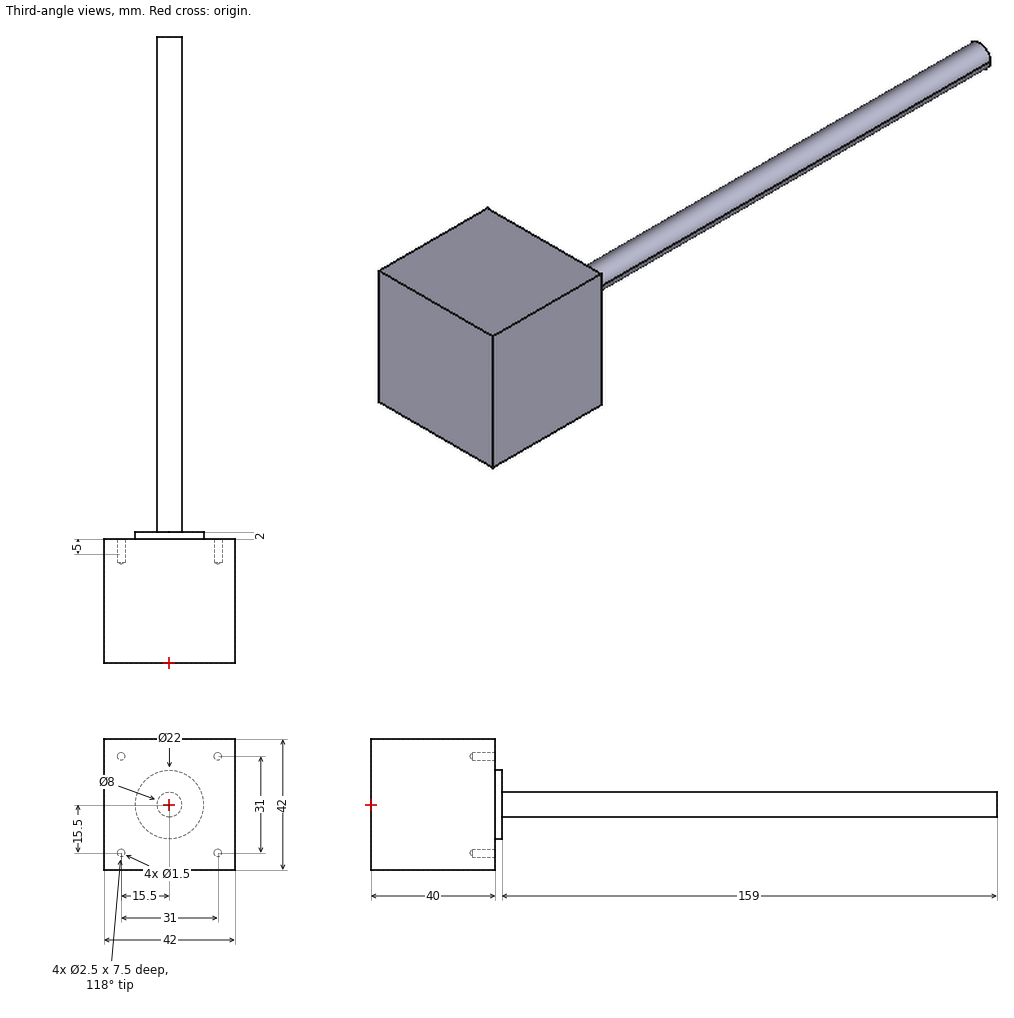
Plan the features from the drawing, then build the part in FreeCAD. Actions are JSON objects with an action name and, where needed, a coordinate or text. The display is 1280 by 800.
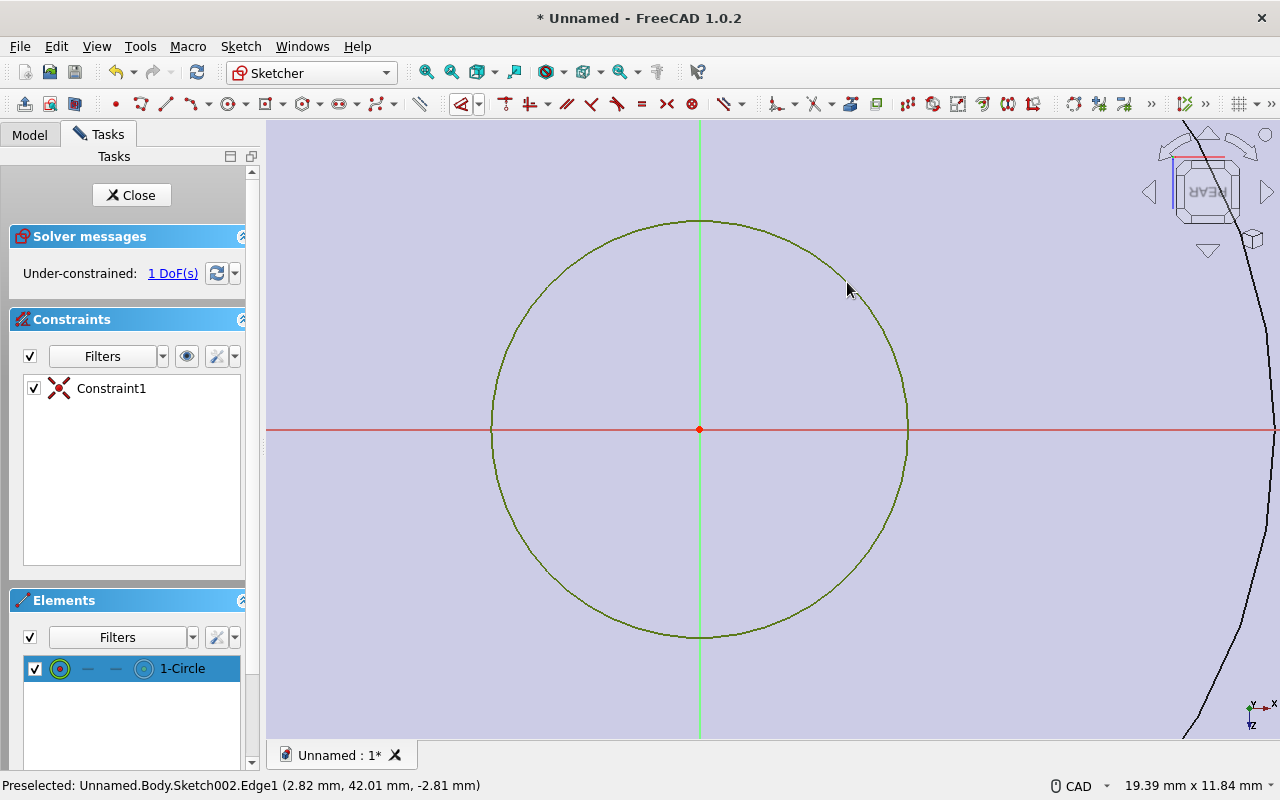
{"action": "key", "text": "k o"}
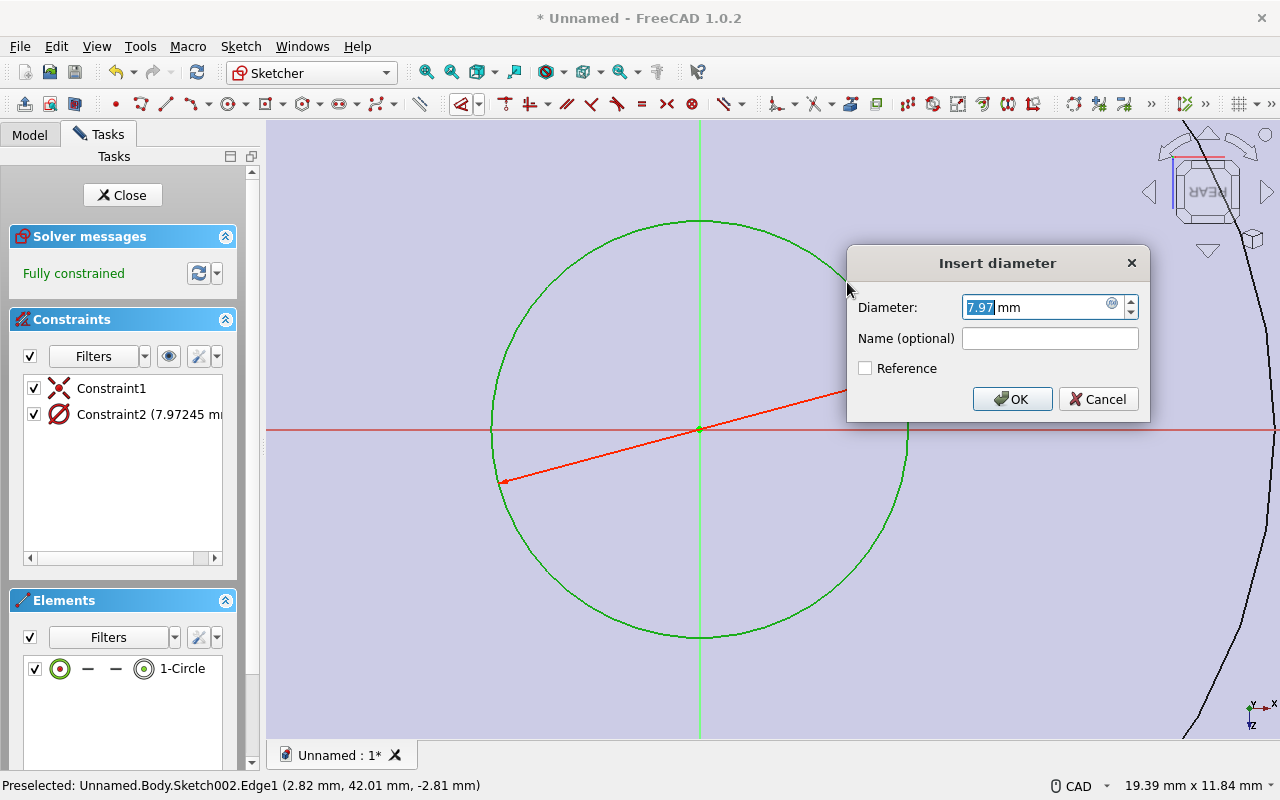
{"action": "type", "text": "8"}
{"action": "key", "text": "Return"}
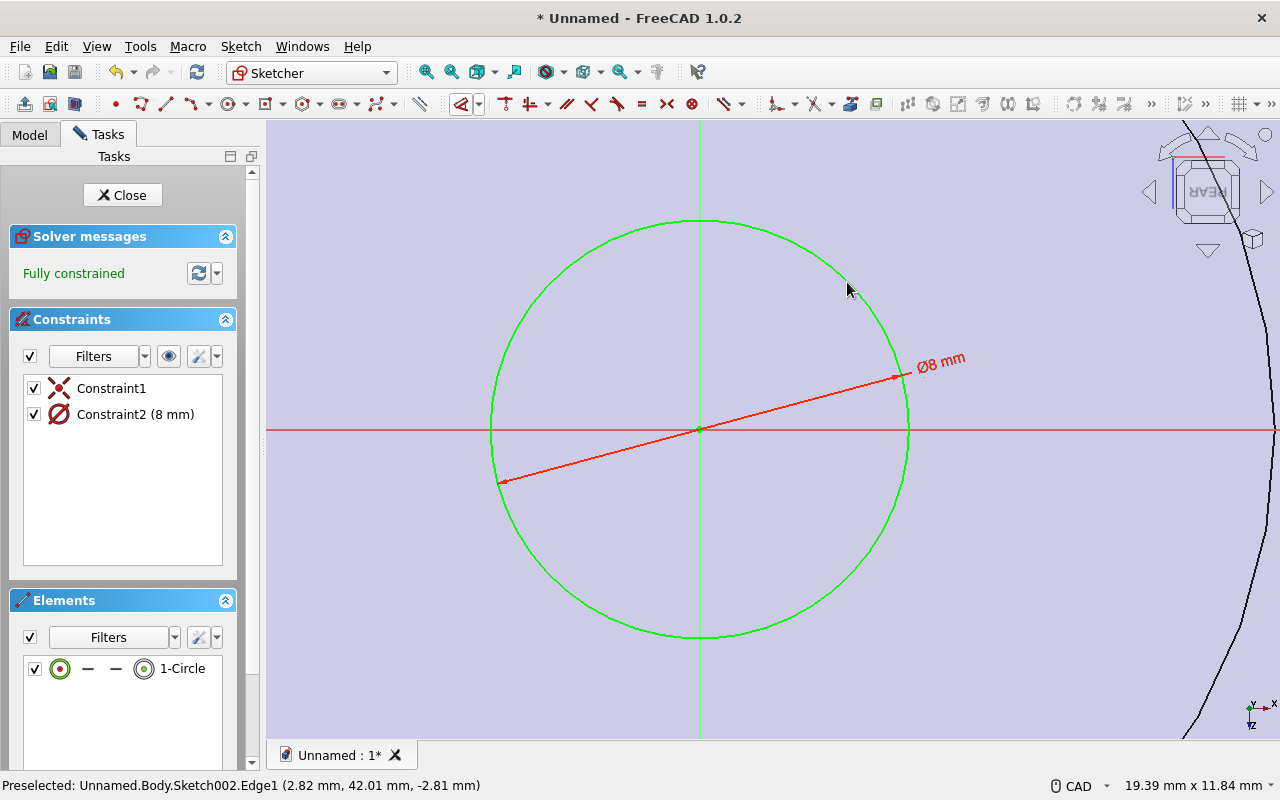
{"action": "left_click", "coordinate": [123, 195]}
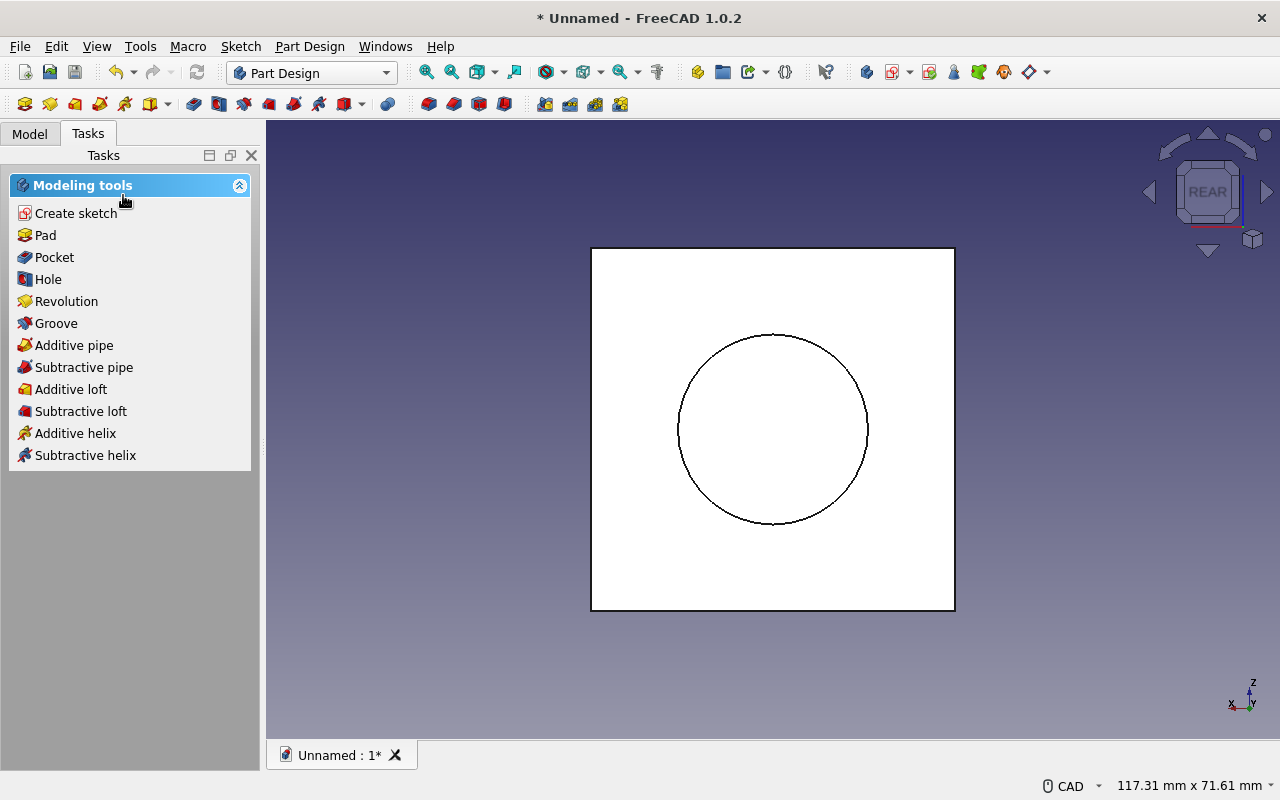
{"action": "left_click", "coordinate": [25, 104]}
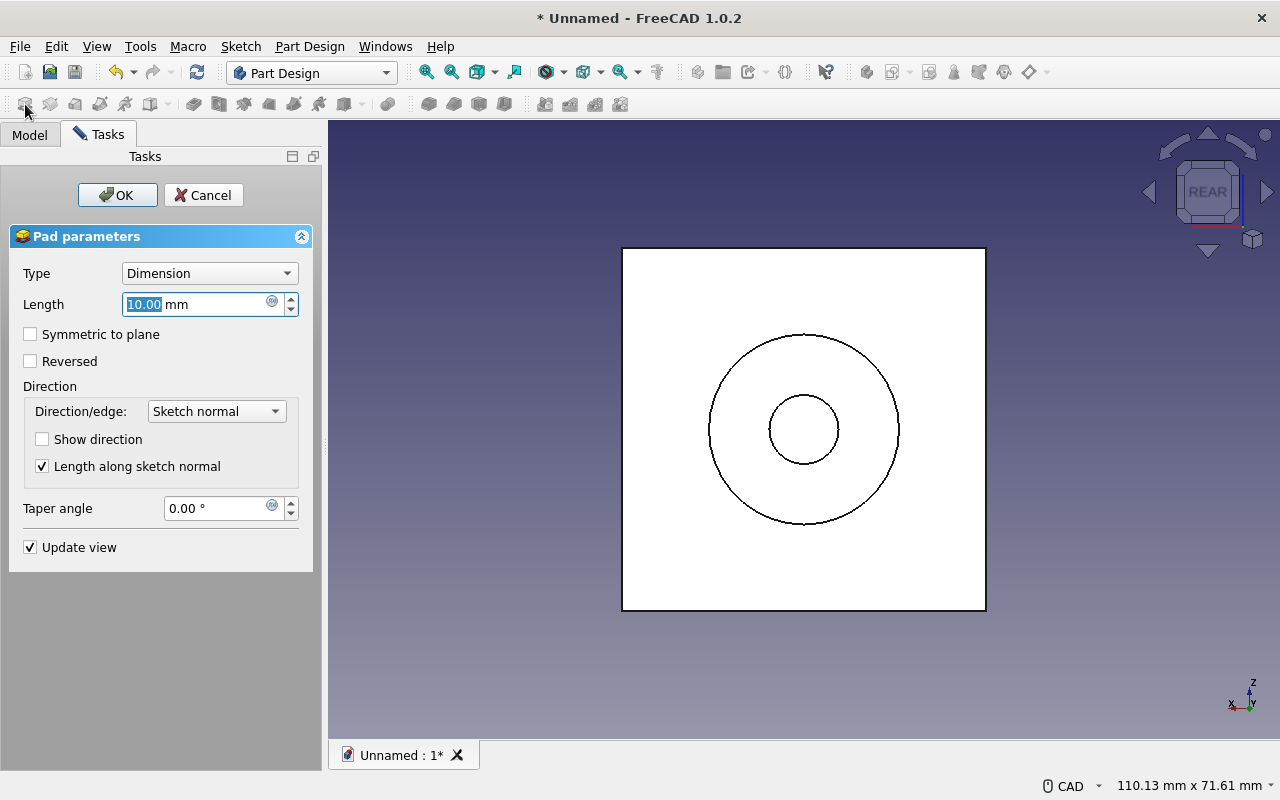
{"action": "type", "text": "159"}
{"action": "key", "text": "Tab"}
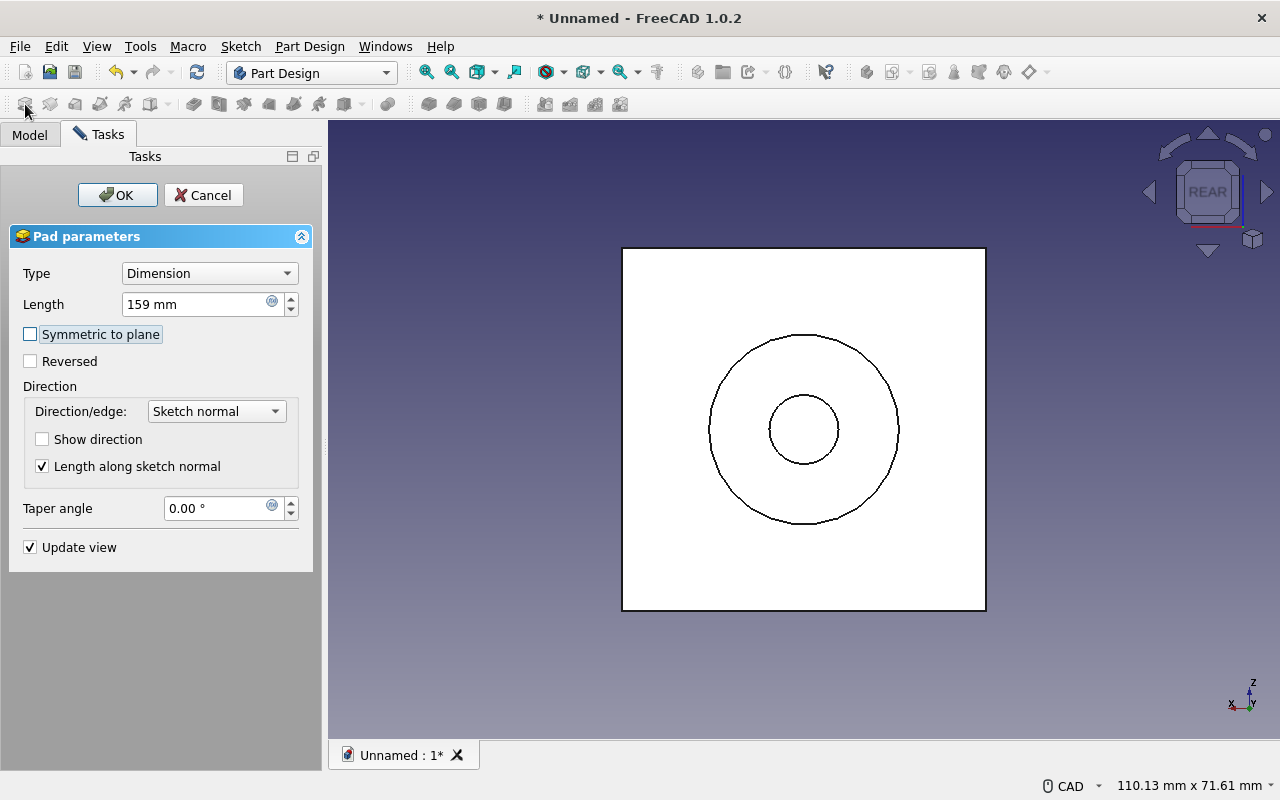
{"action": "left_click", "coordinate": [118, 195]}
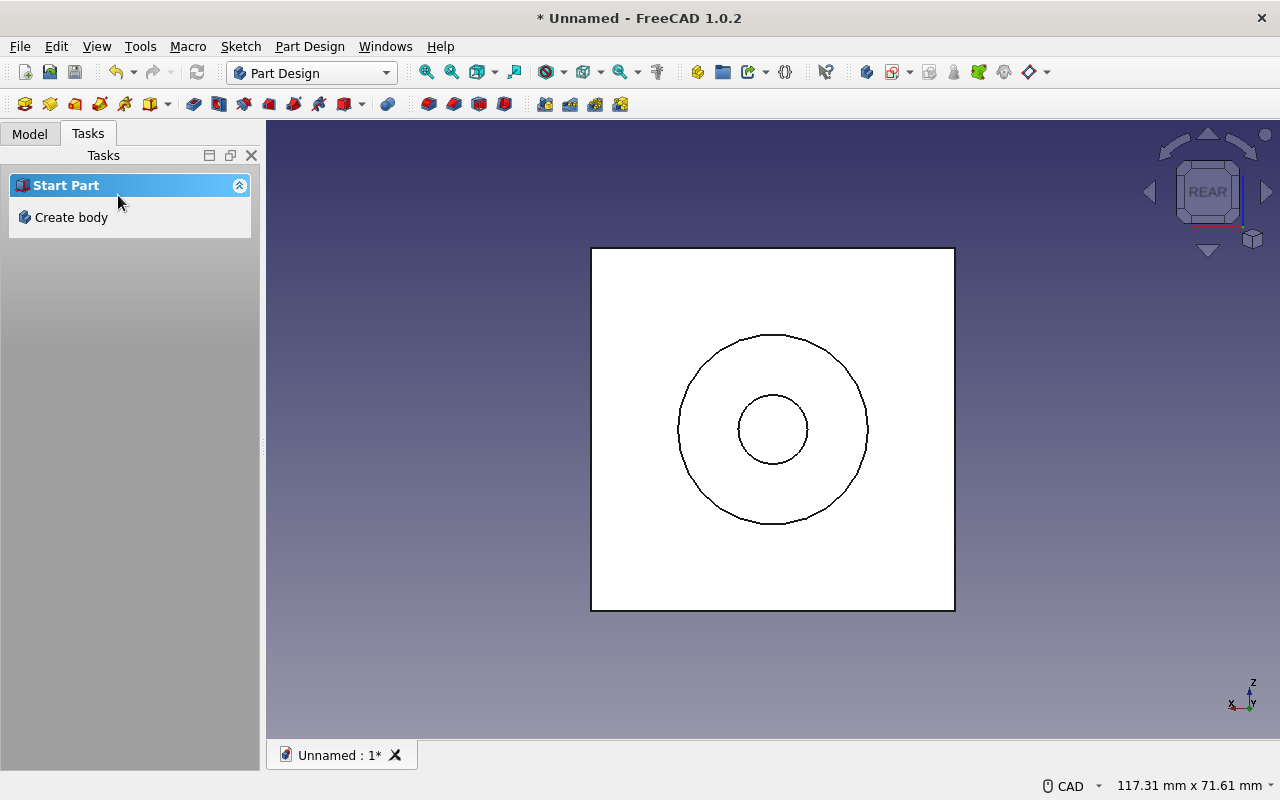
{"action": "left_click", "coordinate": [669, 532]}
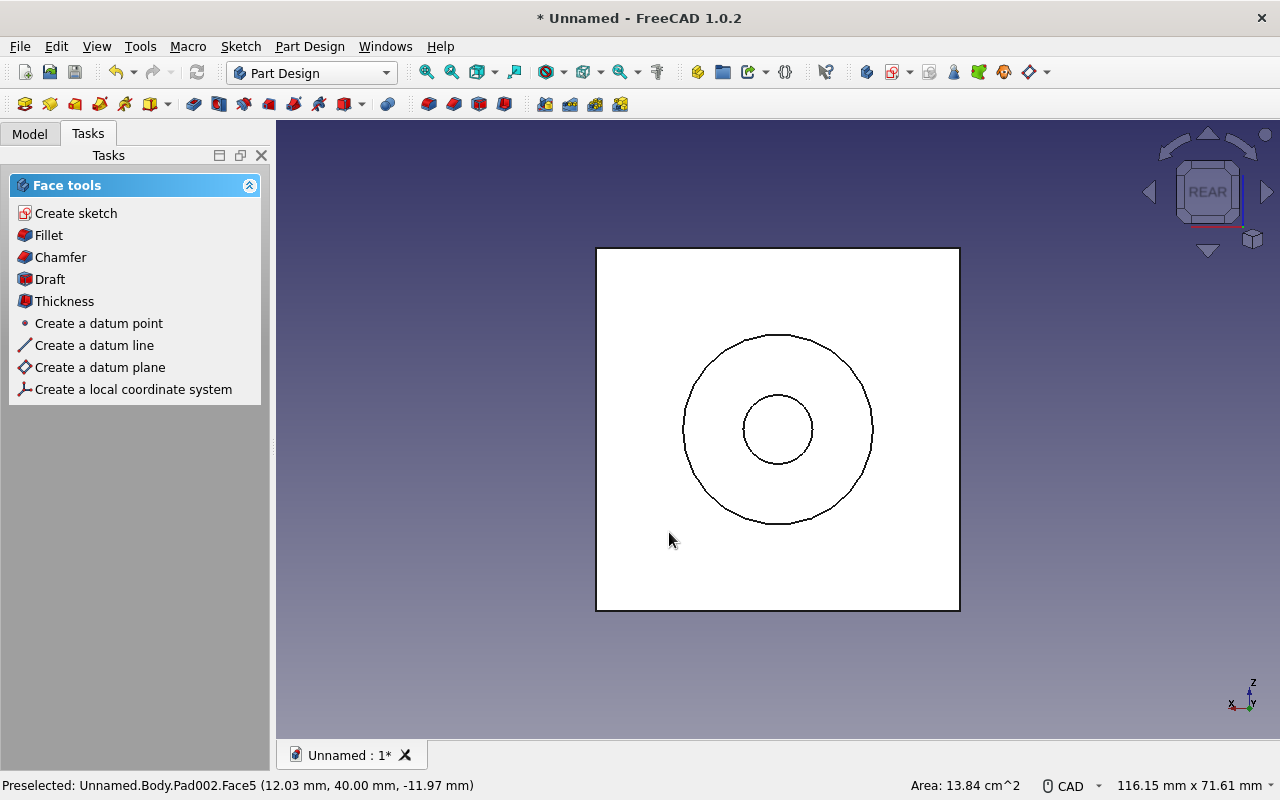
{"action": "left_click", "coordinate": [892, 72]}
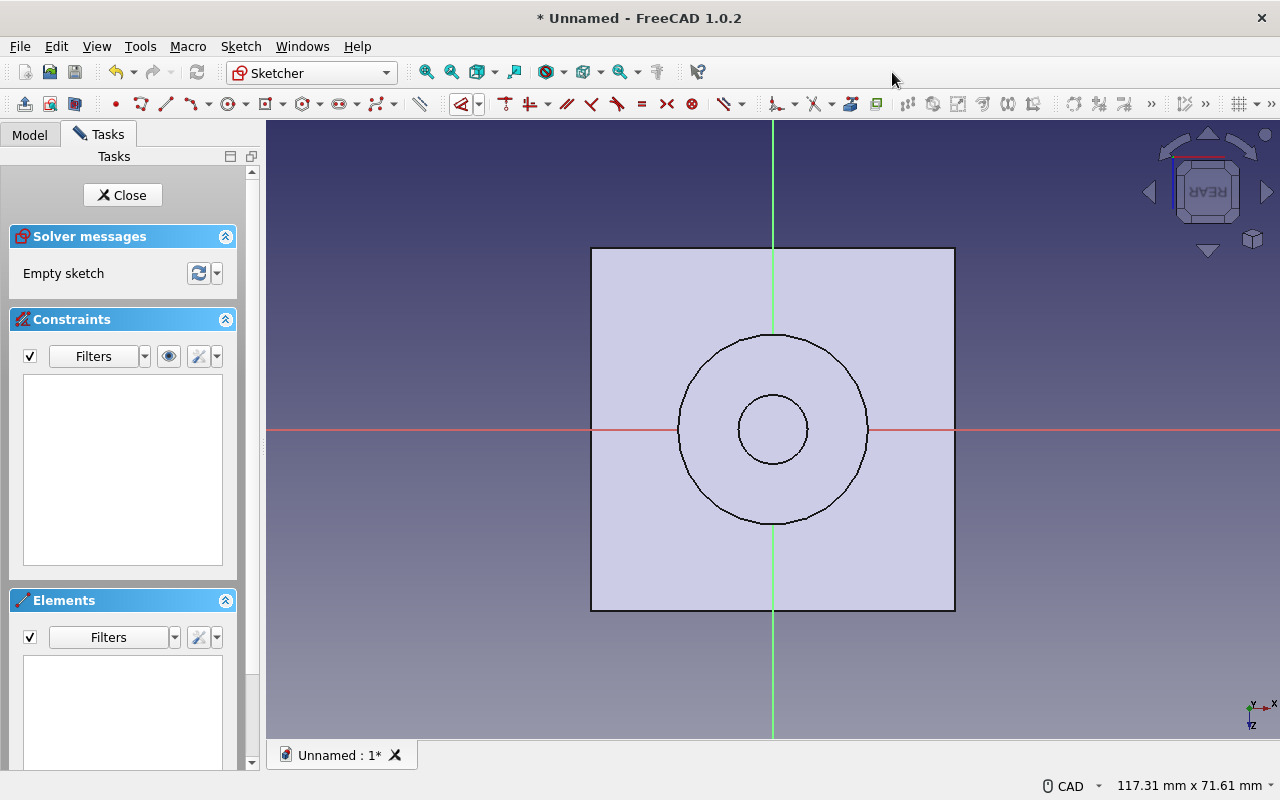
{"action": "scroll", "coordinate": [912, 429], "scroll_direction": "up", "scroll_amount": 2}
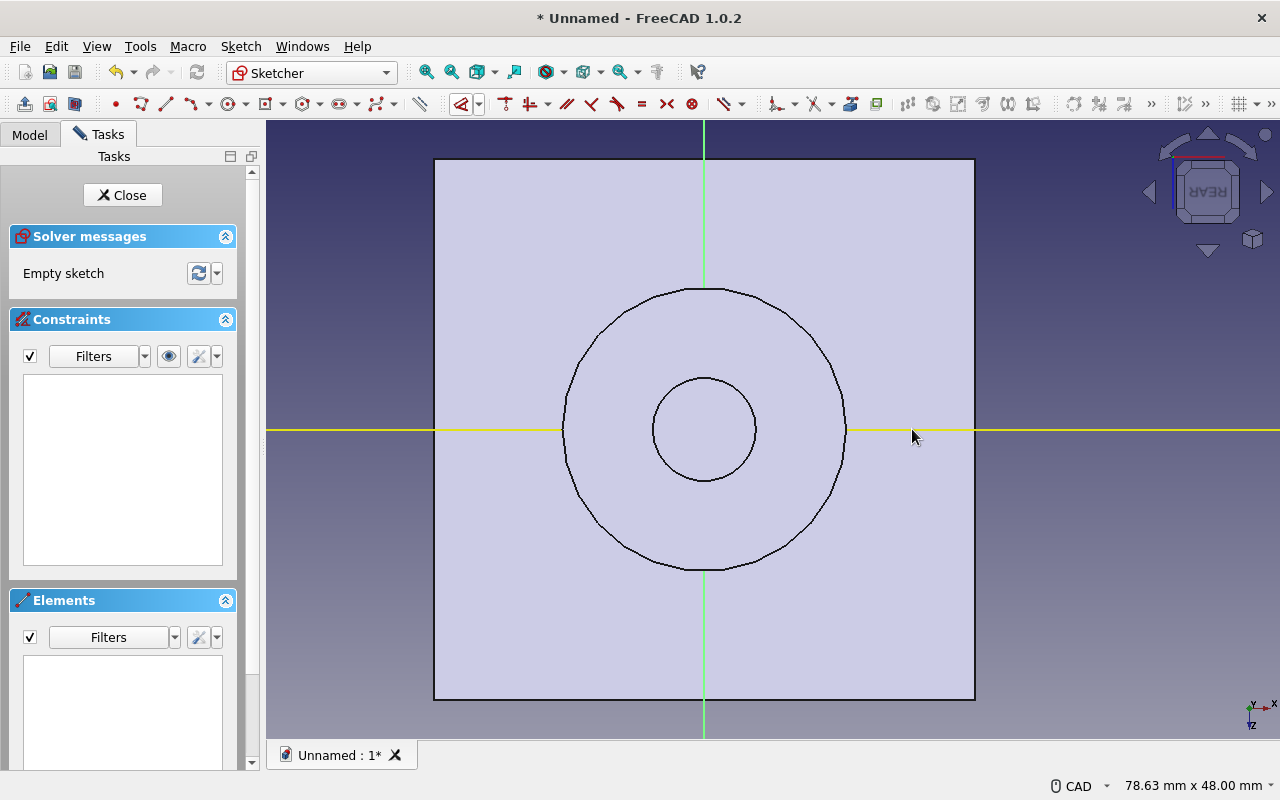
{"action": "left_click", "coordinate": [228, 104]}